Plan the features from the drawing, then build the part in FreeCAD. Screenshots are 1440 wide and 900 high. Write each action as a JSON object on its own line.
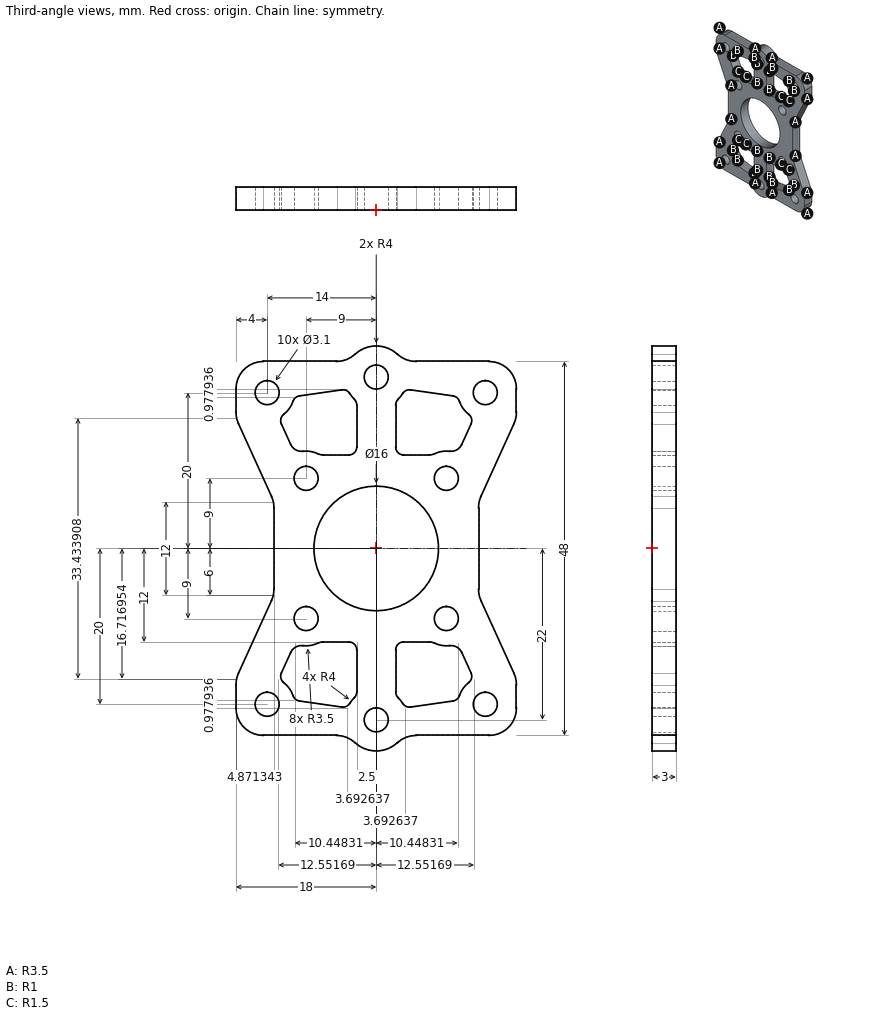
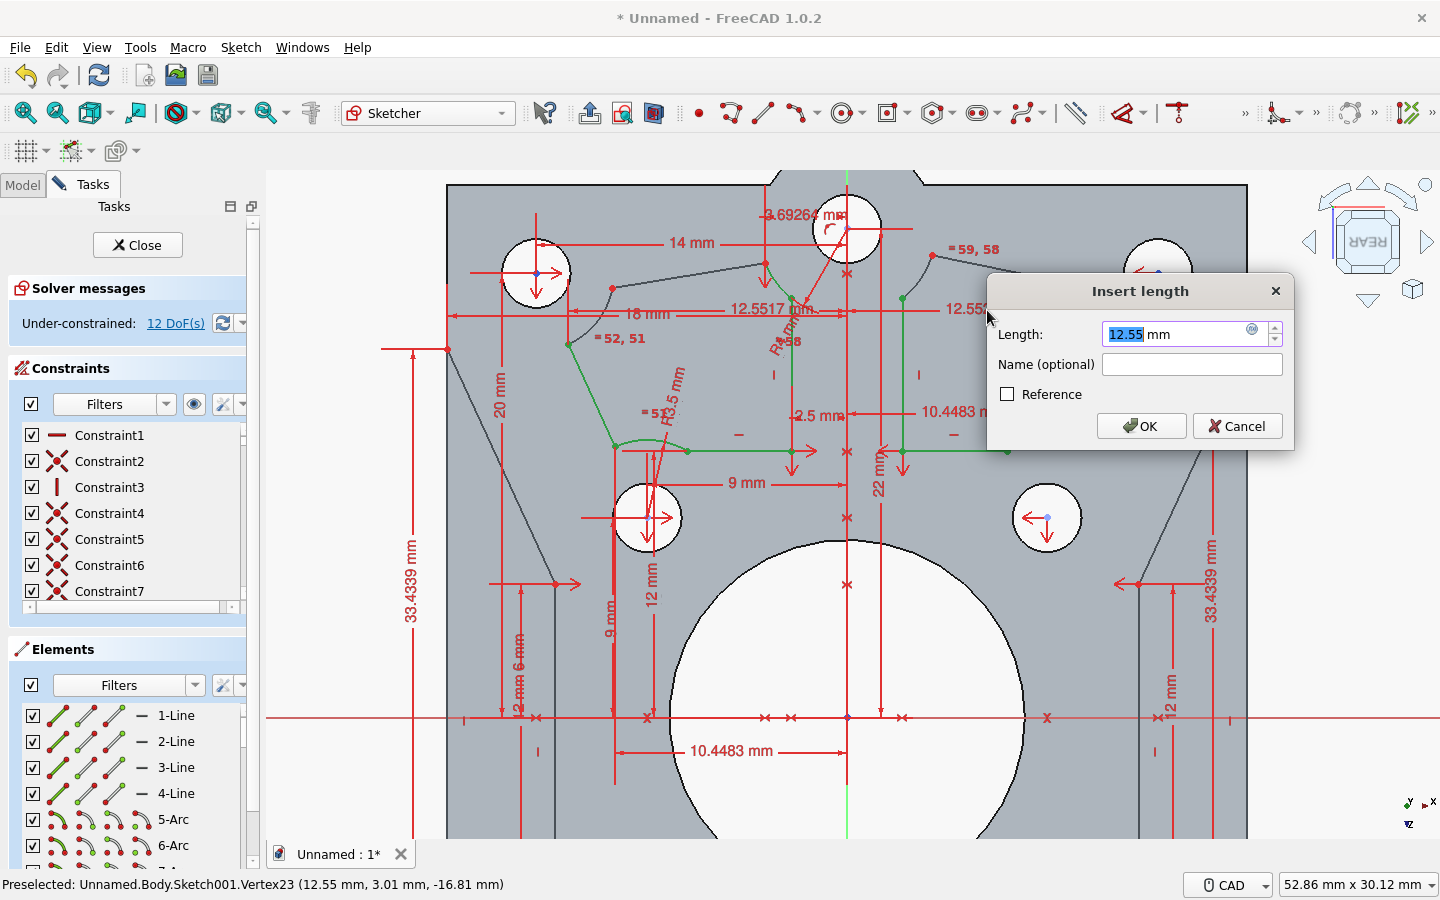
{"action": "type", "text": "12.55169"}
{"action": "key", "text": "Return"}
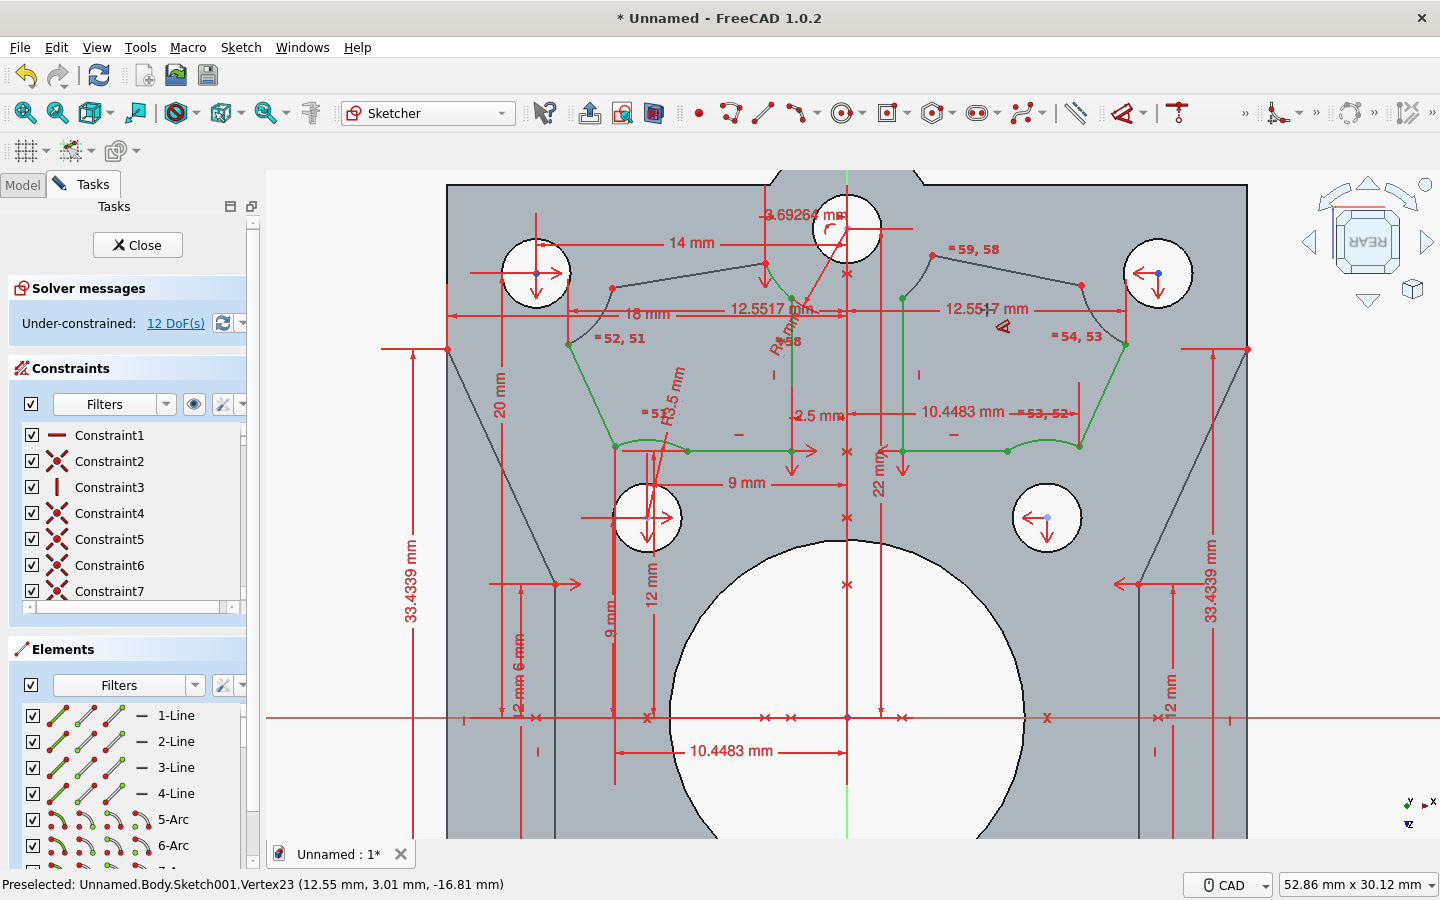
{"action": "left_click", "coordinate": [932, 255]}
{"action": "left_click", "coordinate": [890, 221]}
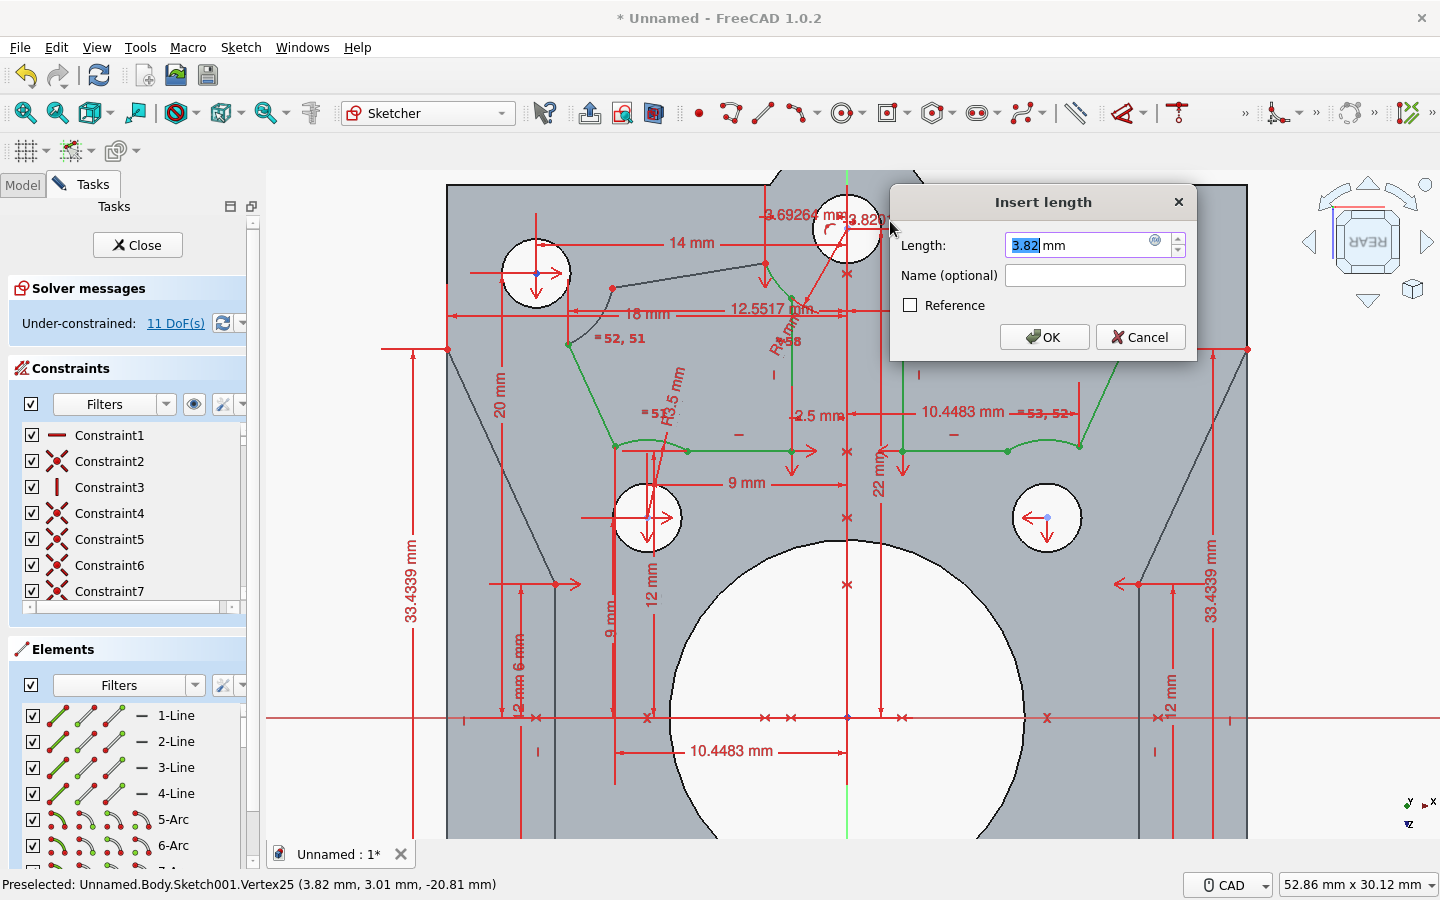
{"action": "type", "text": "3.692637"}
{"action": "key", "text": "Return"}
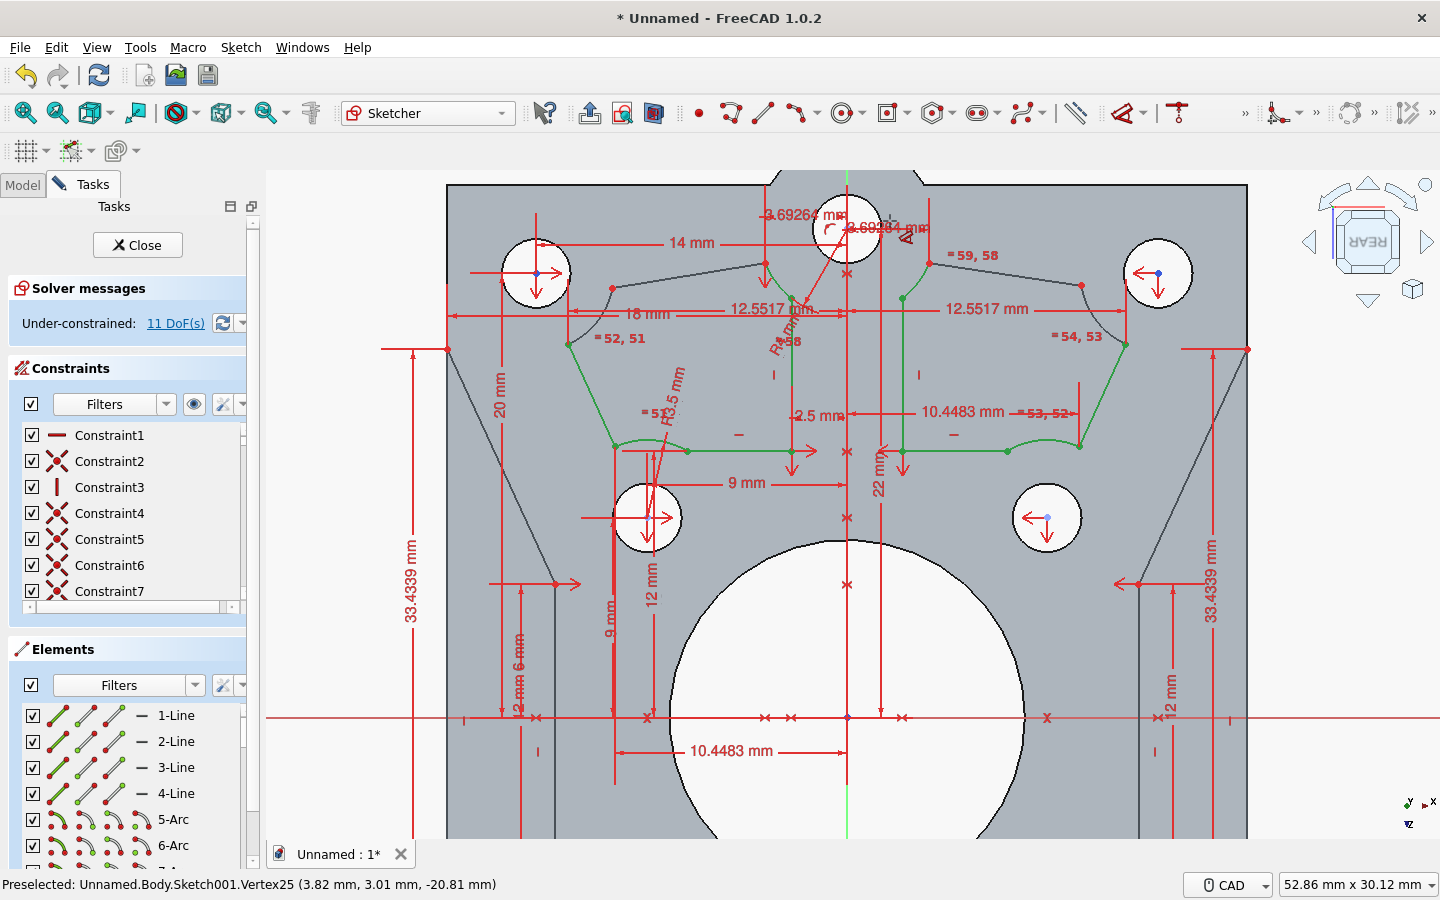
{"action": "scroll", "coordinate": [733, 331], "scroll_direction": "down", "scroll_amount": 4}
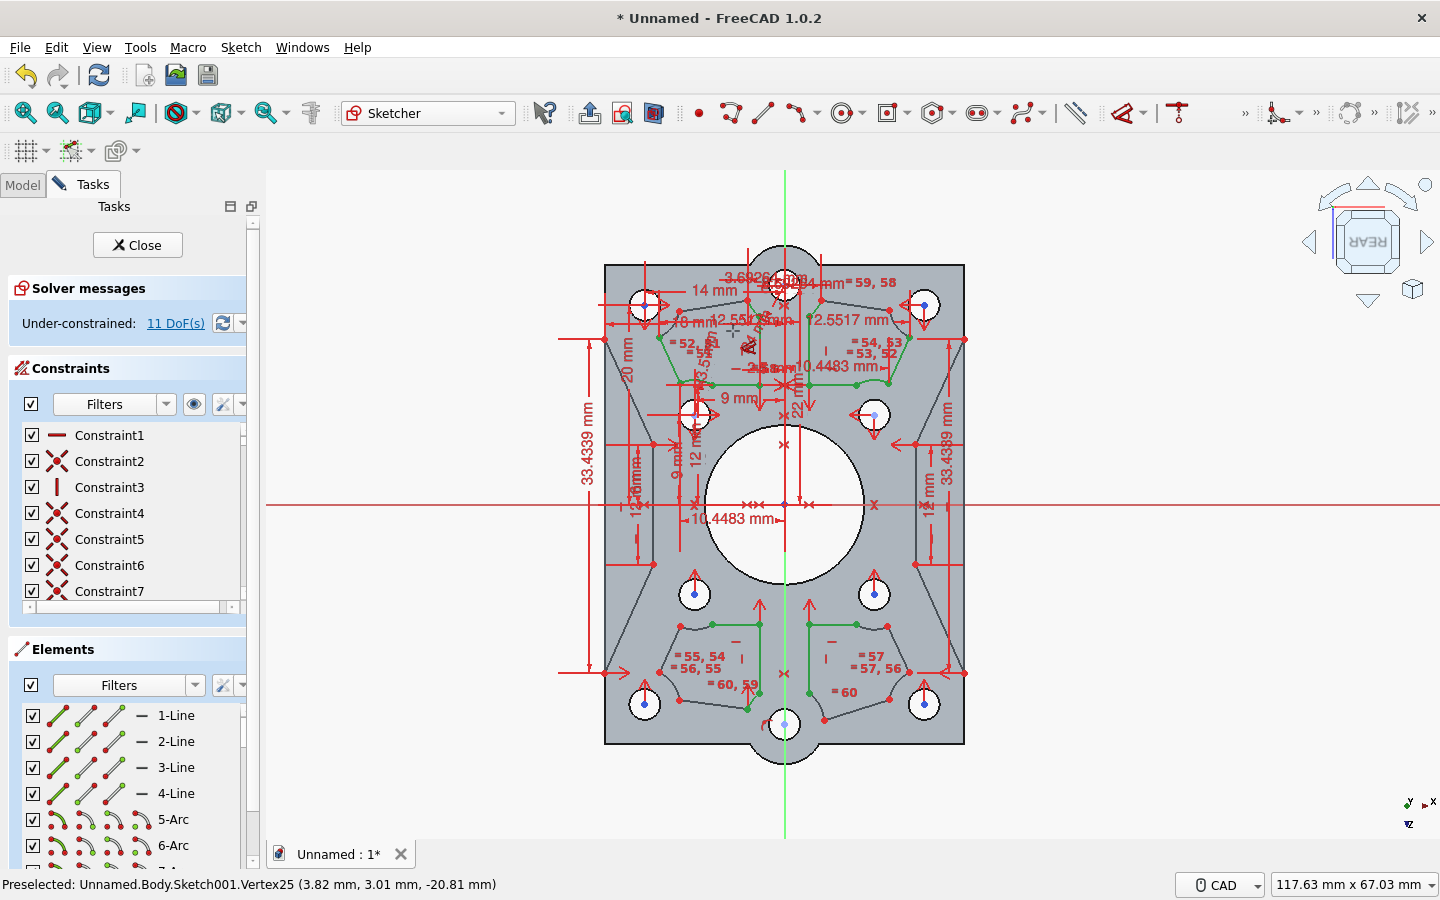
{"action": "left_click", "coordinate": [680, 627]}
{"action": "left_click", "coordinate": [732, 661]}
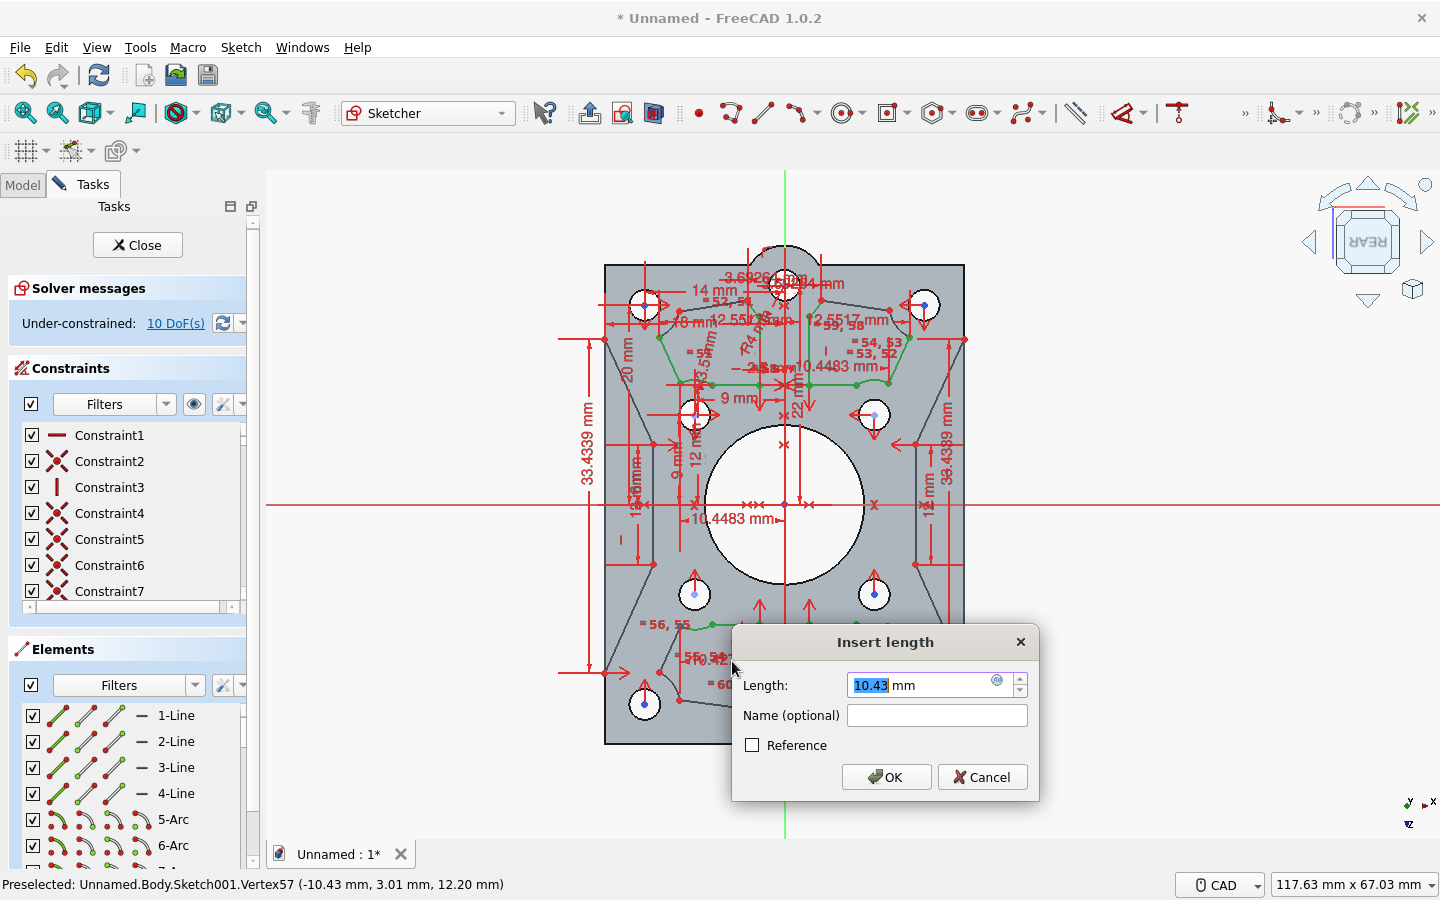
{"action": "type", "text": "10.44831"}
{"action": "key", "text": "Return"}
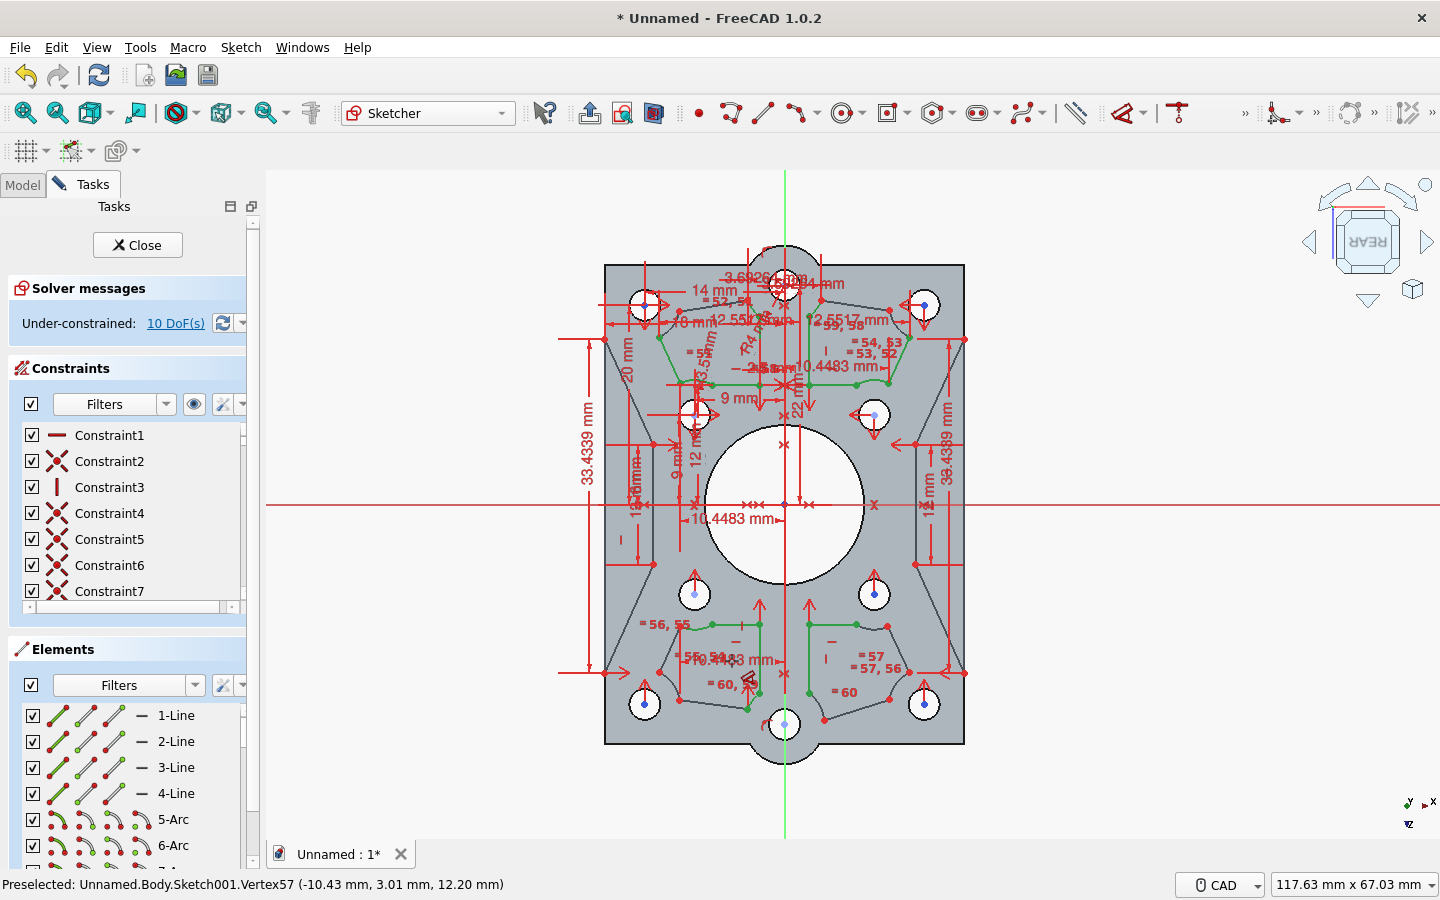
{"action": "left_click", "coordinate": [660, 673]}
{"action": "left_click", "coordinate": [766, 707]}